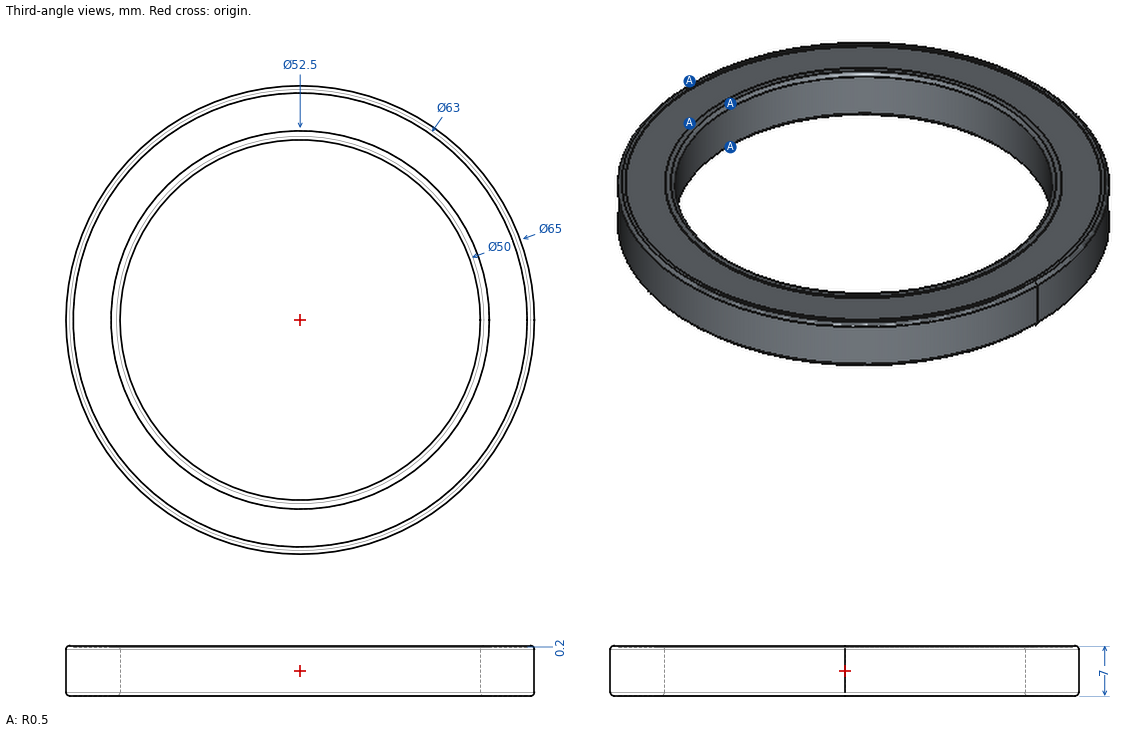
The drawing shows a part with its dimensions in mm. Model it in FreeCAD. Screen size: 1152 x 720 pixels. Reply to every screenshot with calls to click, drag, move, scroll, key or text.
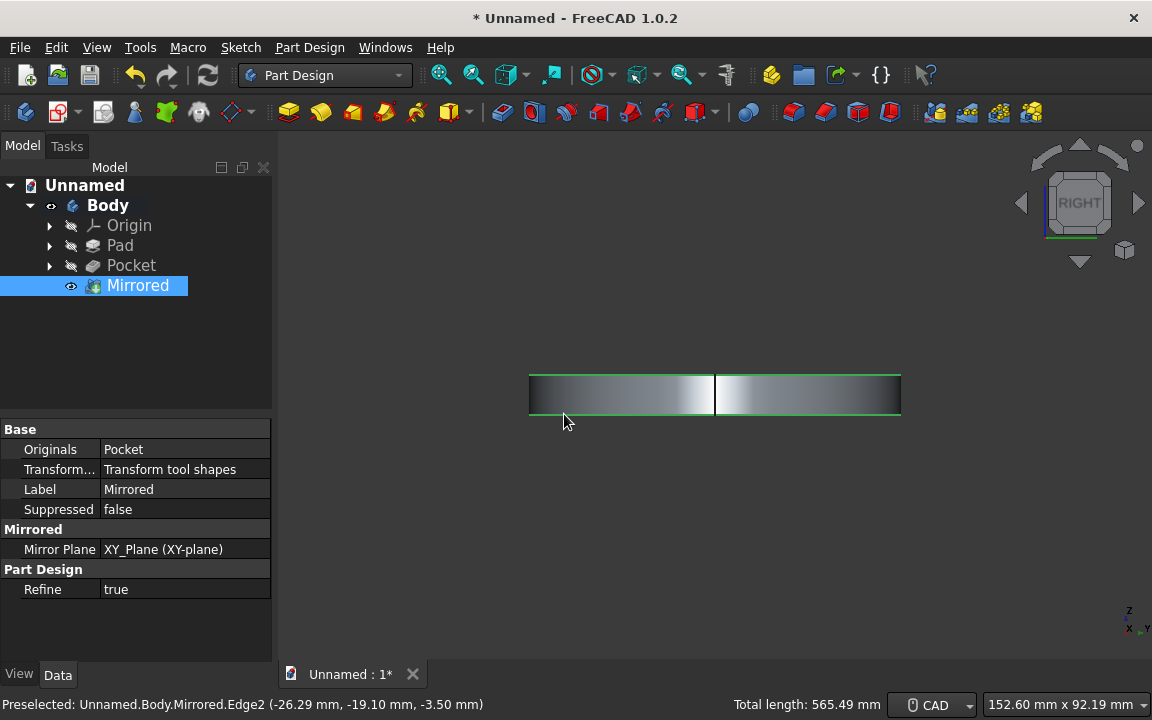
key(5)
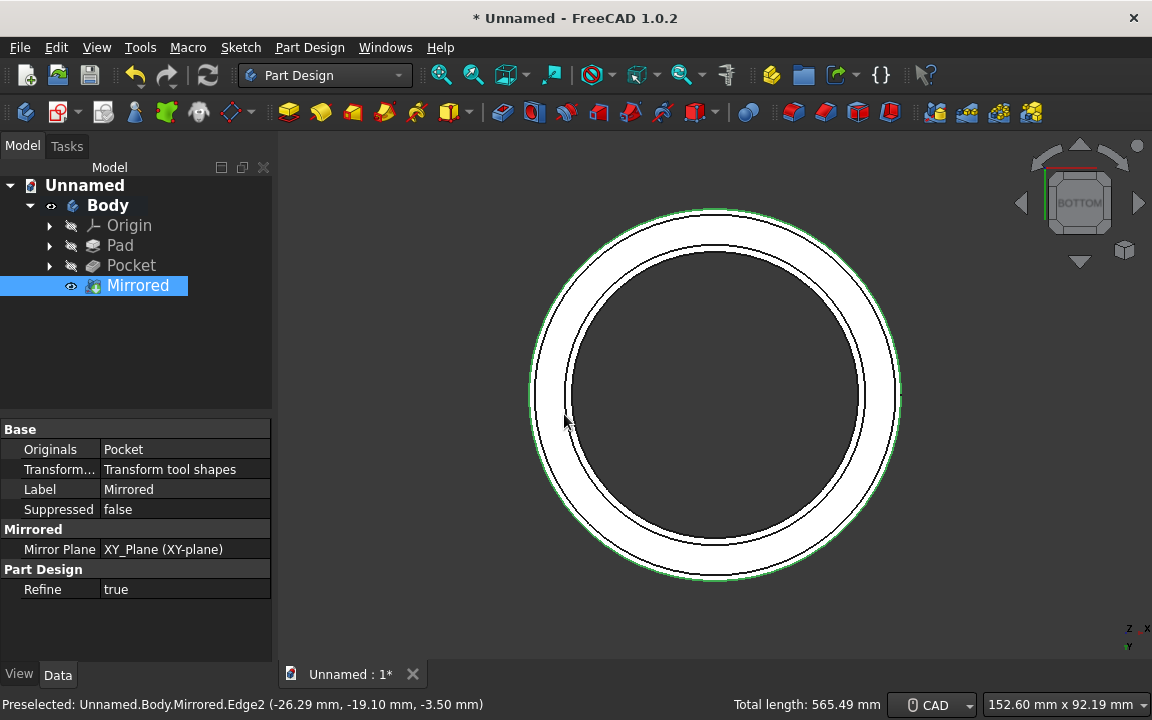
click(572, 394, ctrl)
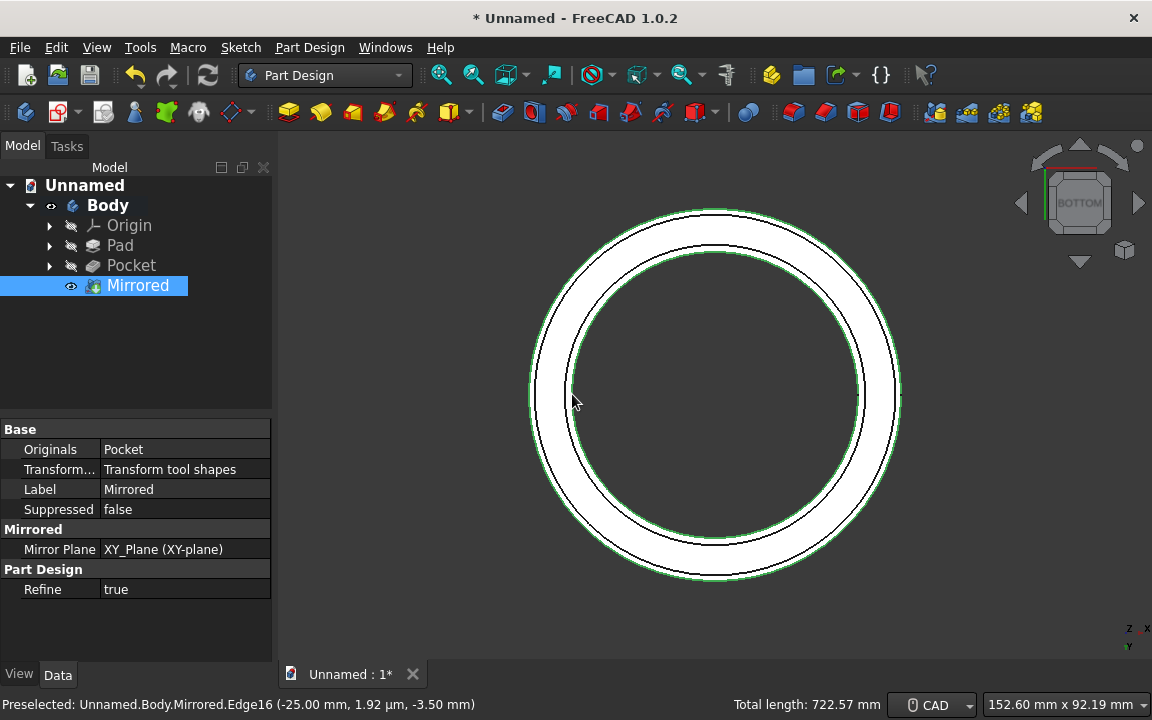
click(794, 112)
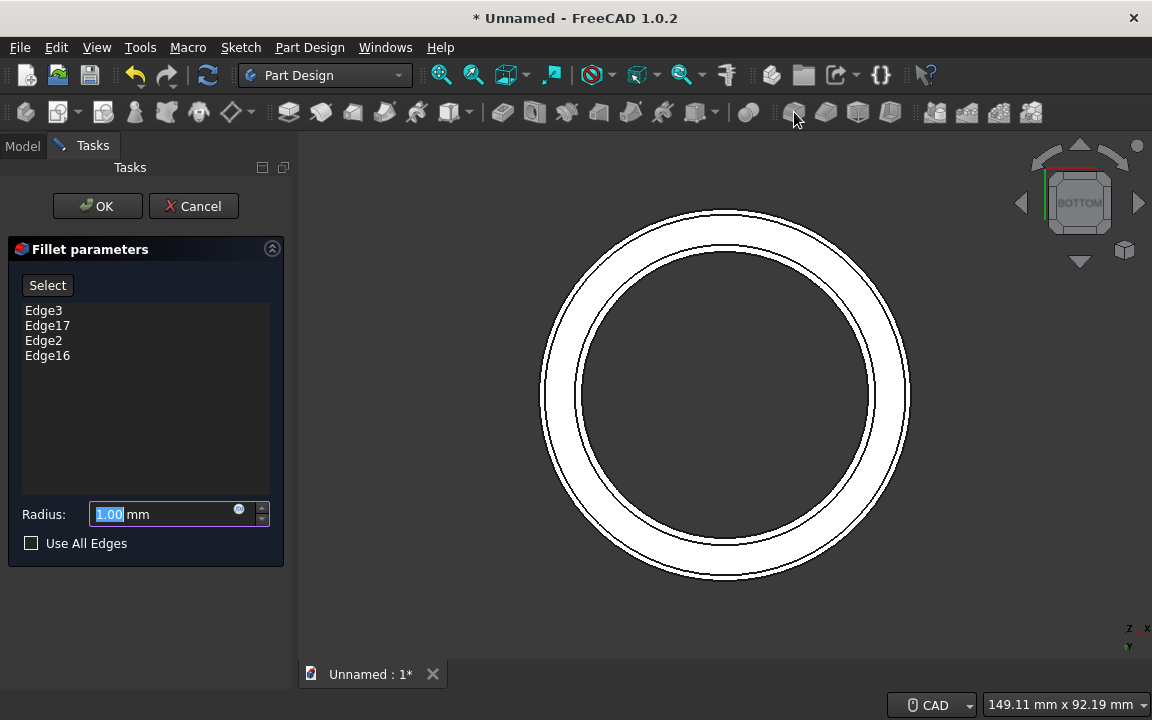
text(0.5)
key(Tab)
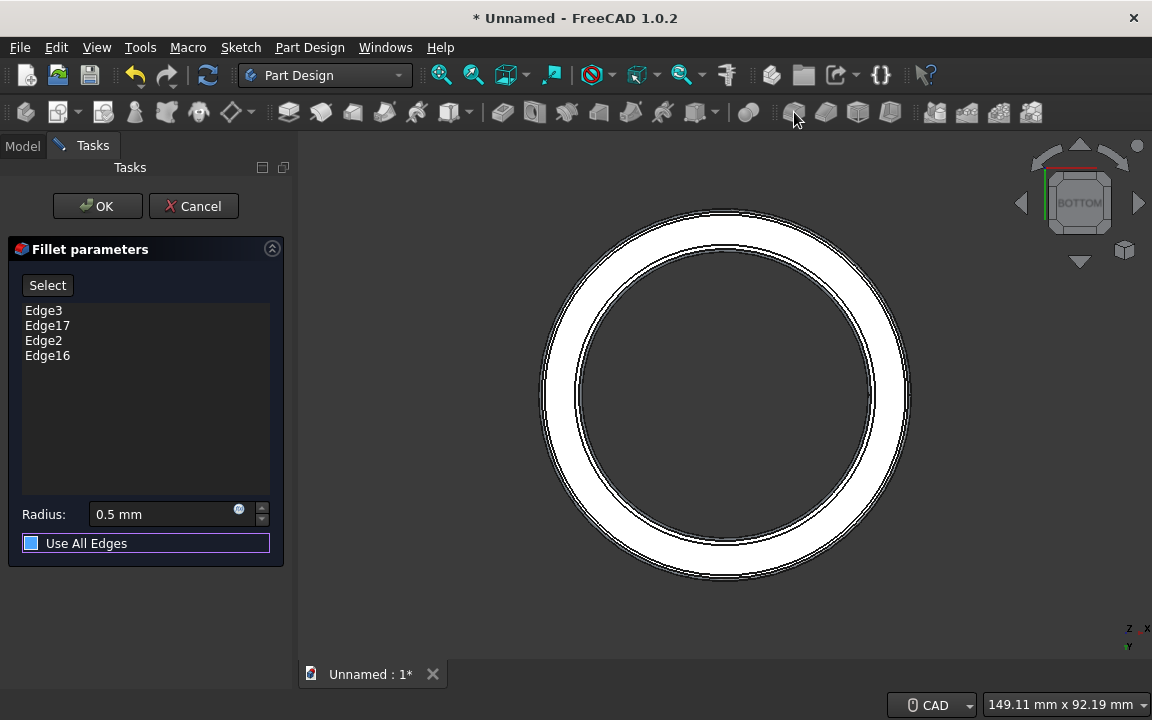
click(98, 206)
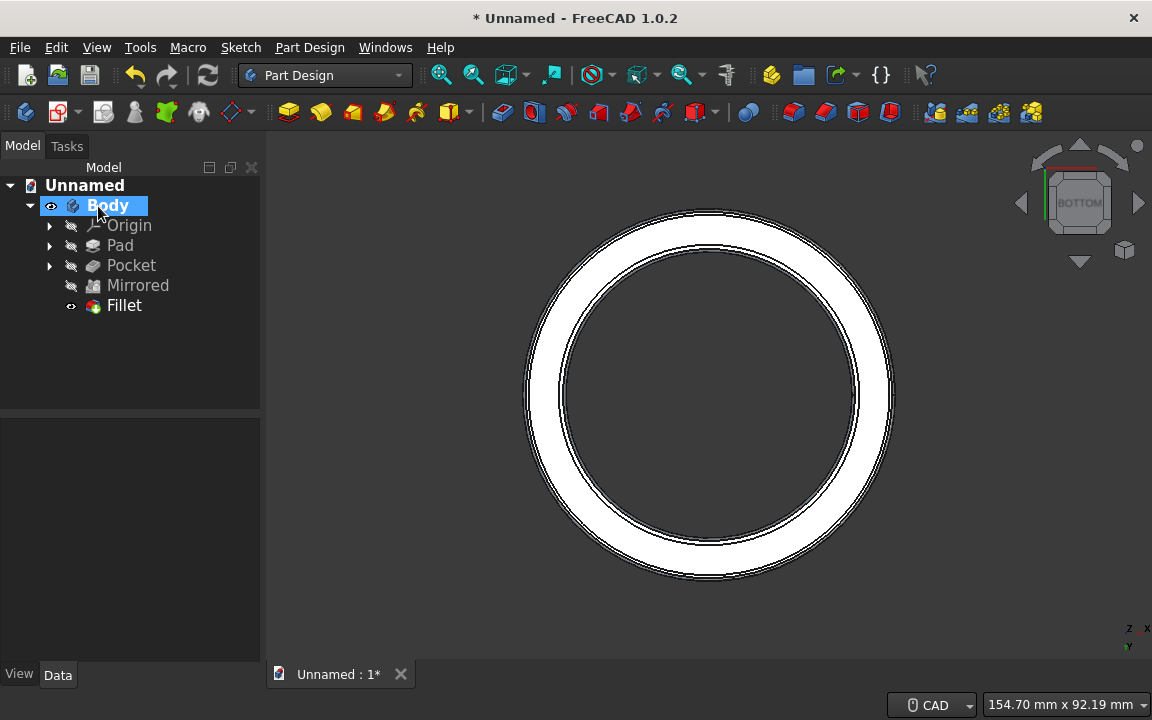
key(0)